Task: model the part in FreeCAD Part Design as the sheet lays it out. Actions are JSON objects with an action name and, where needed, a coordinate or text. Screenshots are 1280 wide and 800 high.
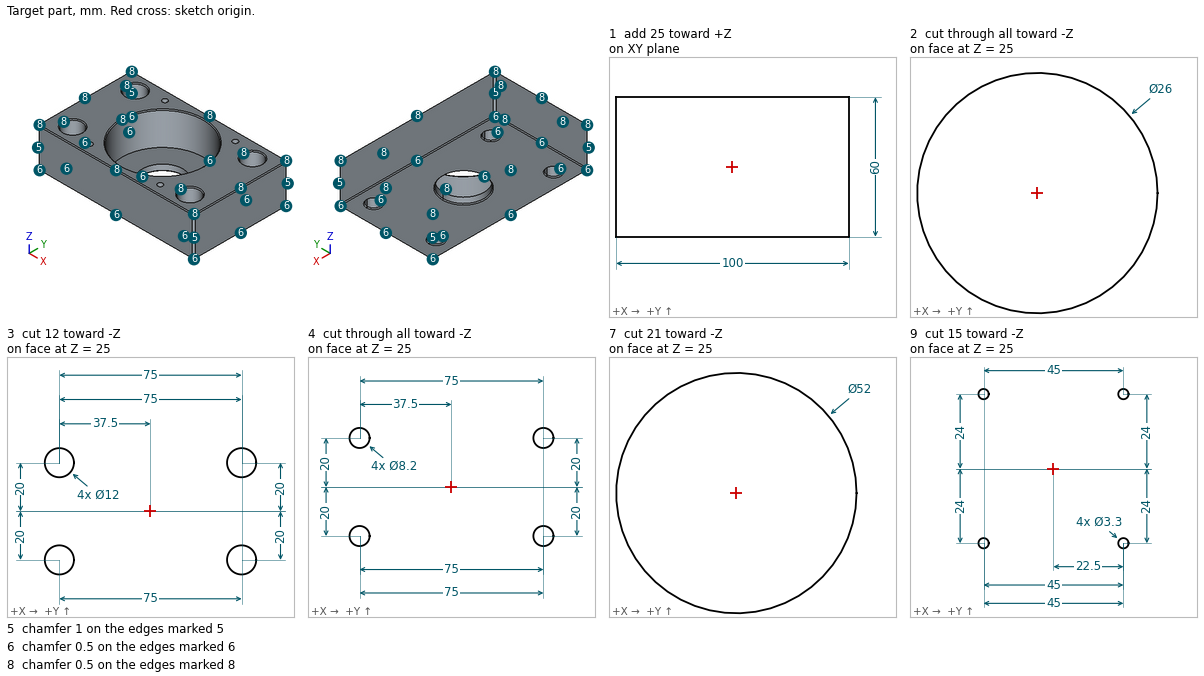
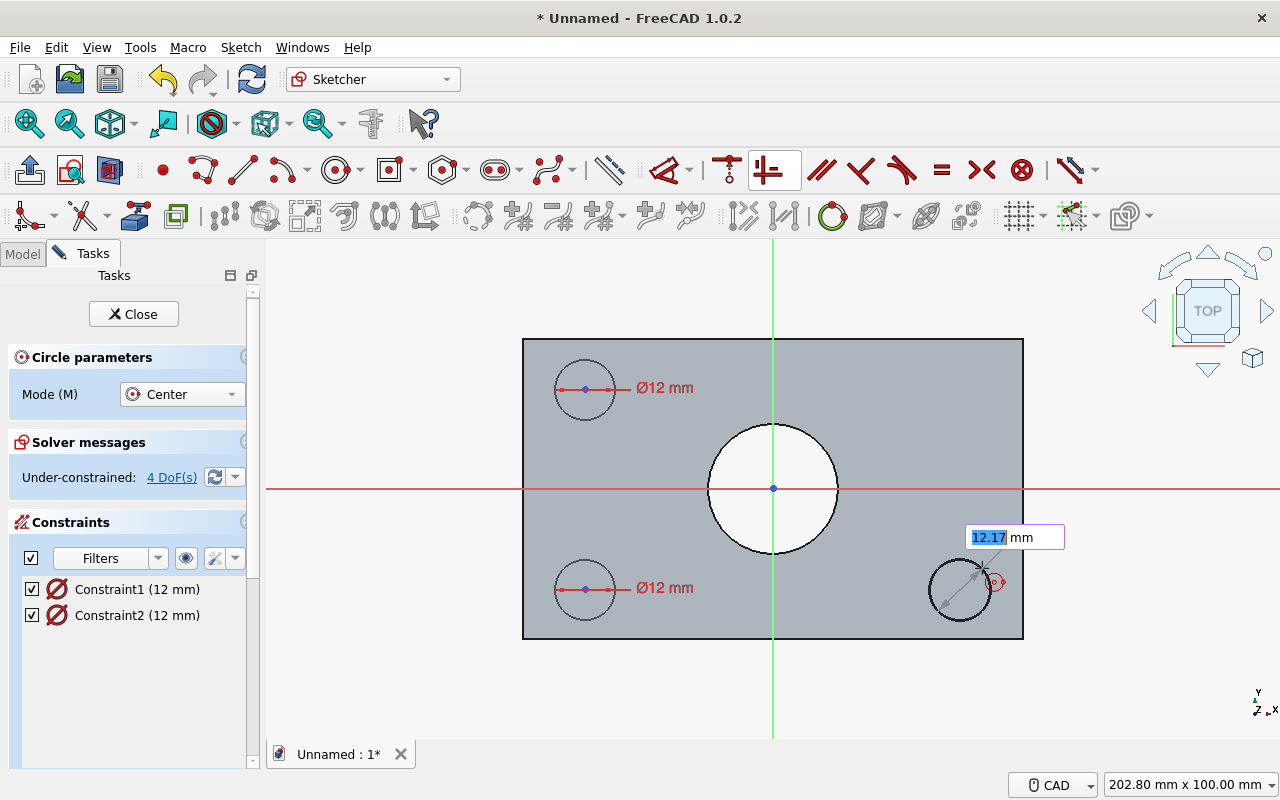
{"action": "type", "text": "12"}
{"action": "key", "text": "Return"}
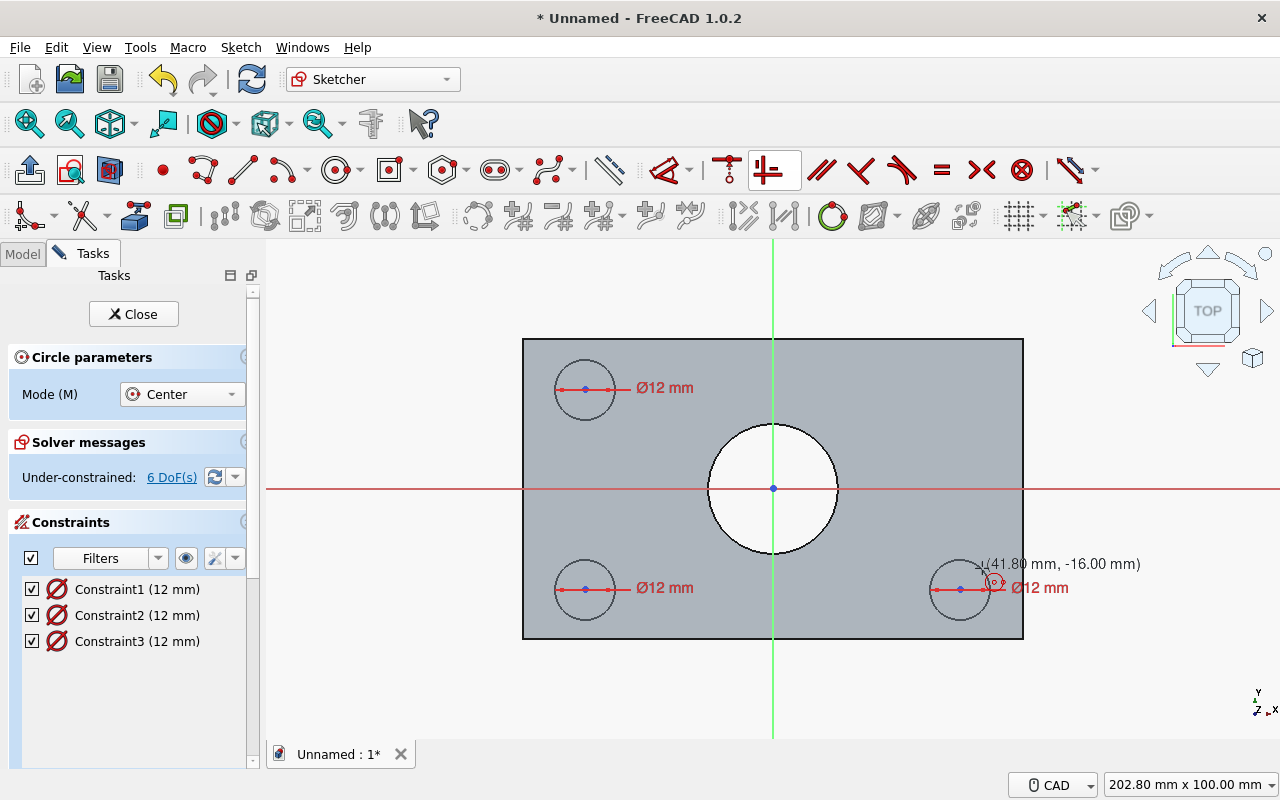
{"action": "left_click", "coordinate": [960, 389]}
{"action": "mouse_move", "coordinate": [982, 368]}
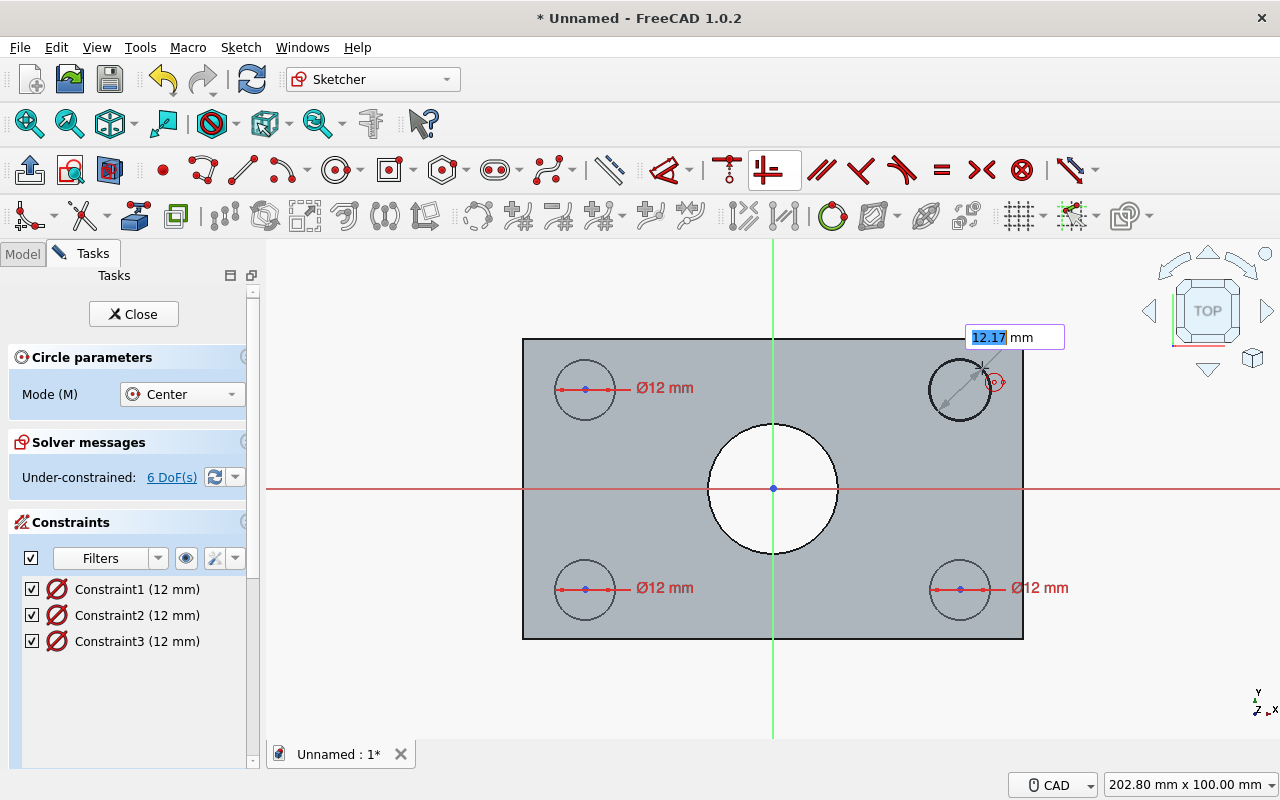
{"action": "type", "text": "12"}
{"action": "key", "text": "Return"}
{"action": "key", "text": "Escape"}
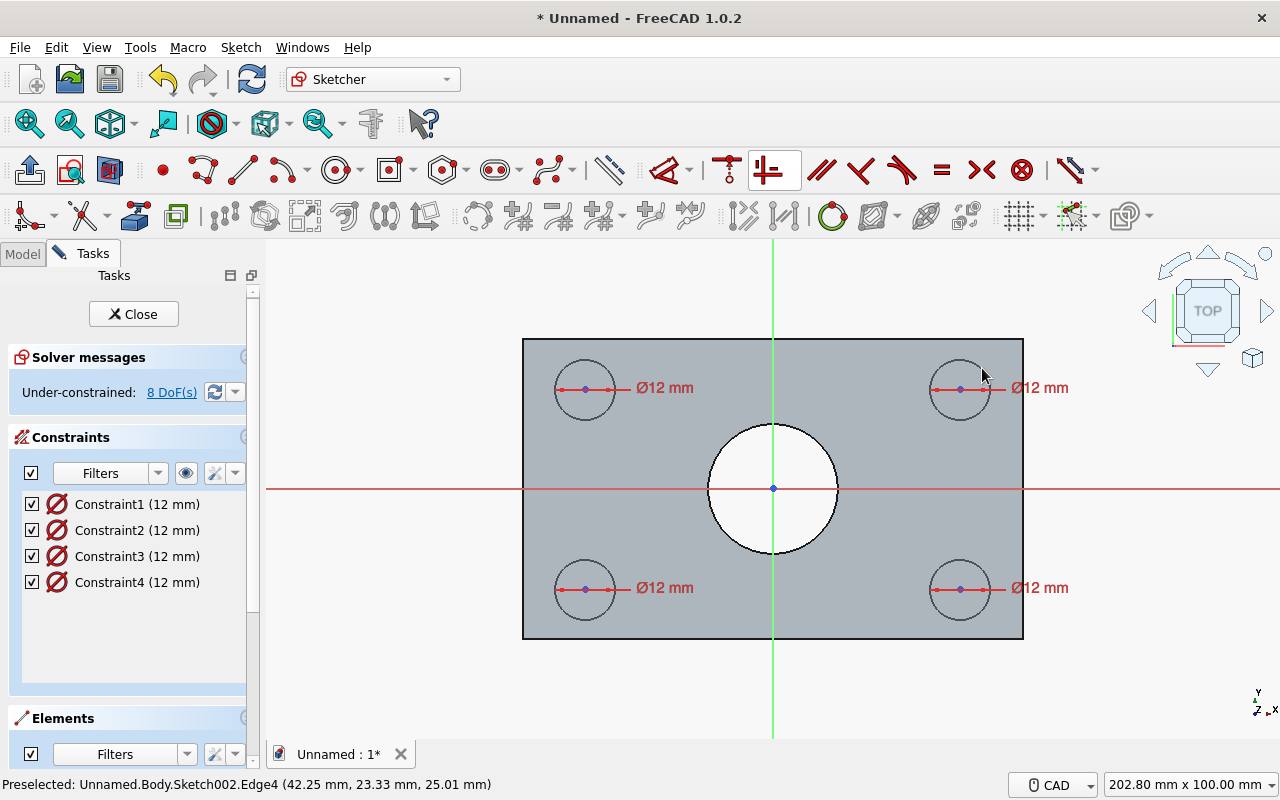
{"action": "left_click", "coordinate": [585, 390]}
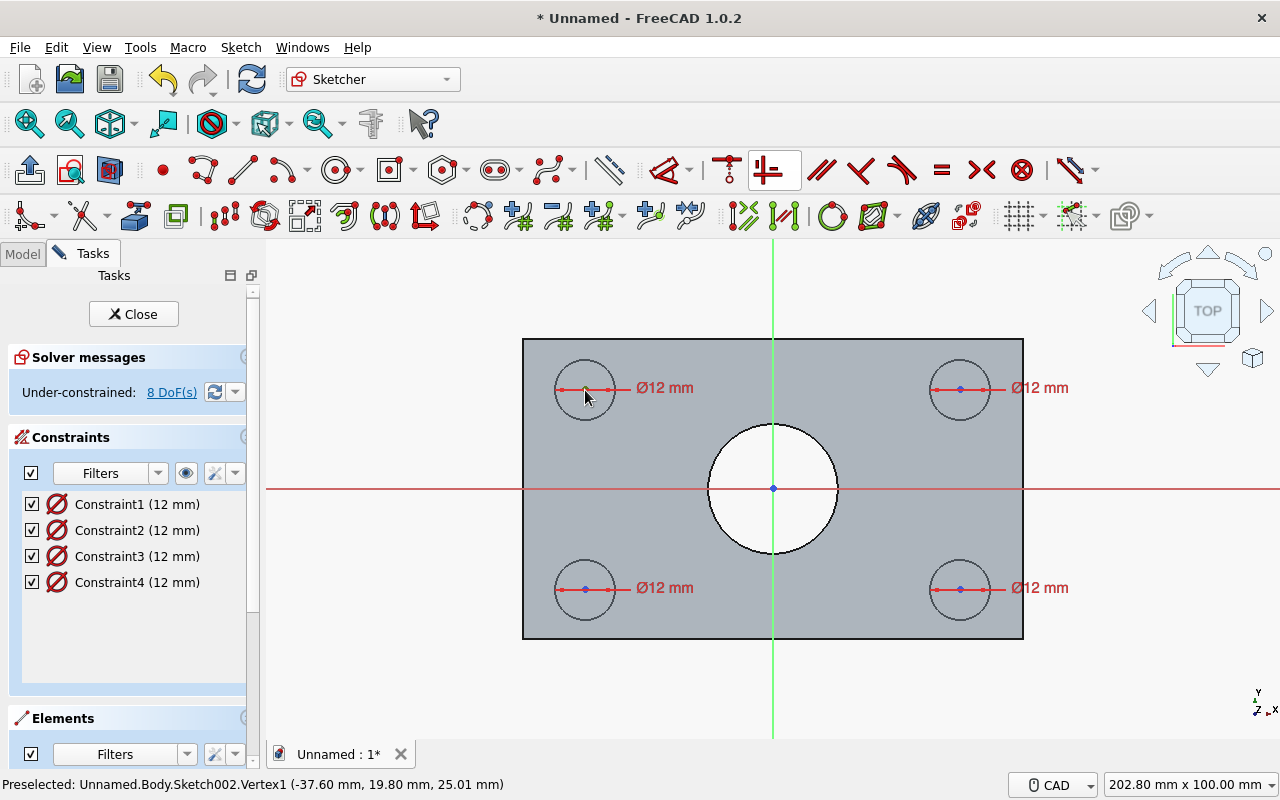
{"action": "key", "text": "i"}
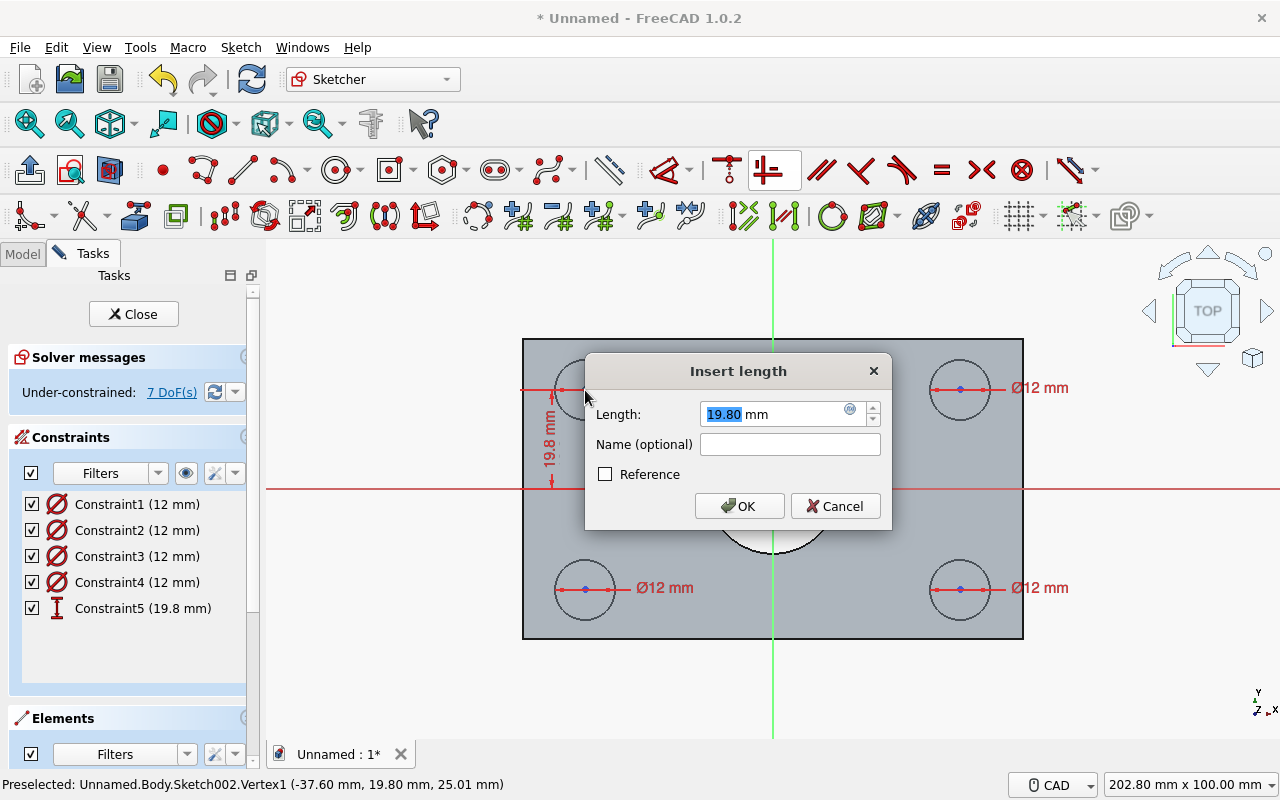
{"action": "type", "text": "20"}
{"action": "key", "text": "Return"}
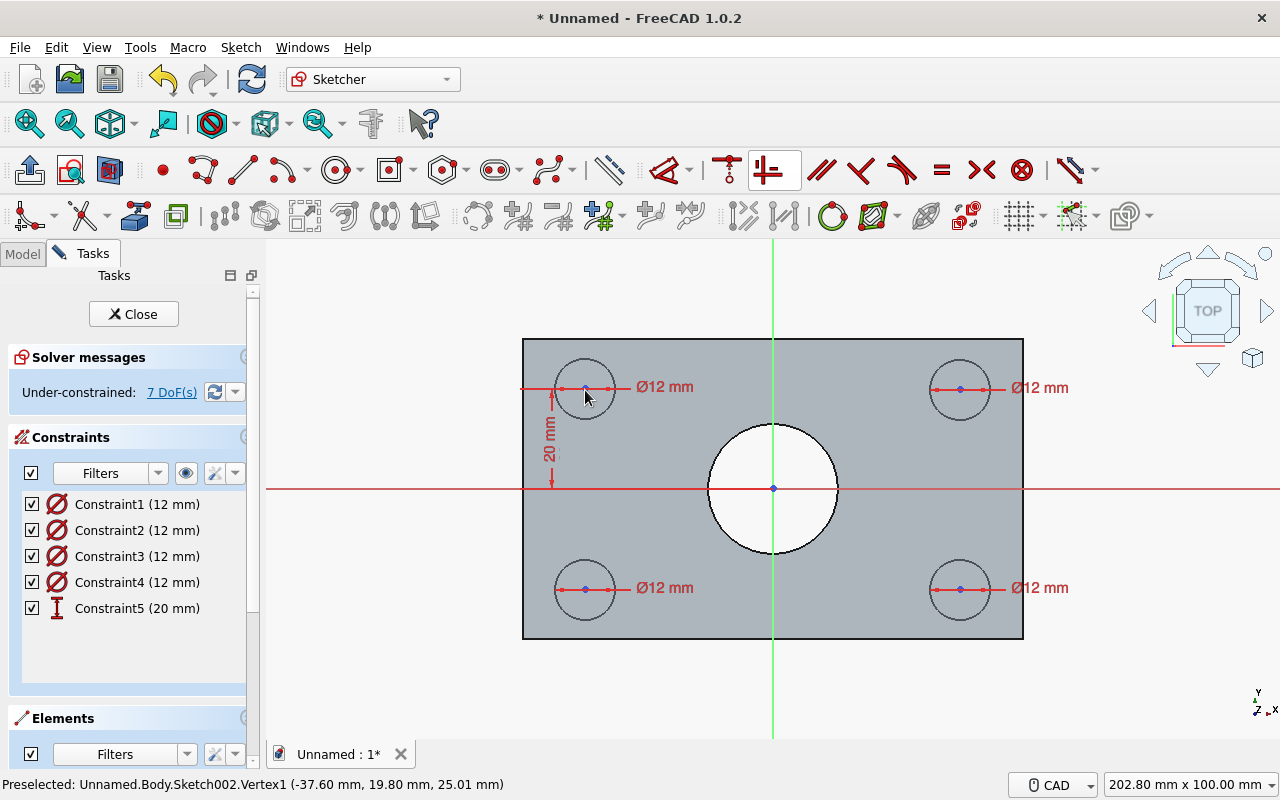
{"action": "left_click", "coordinate": [585, 590]}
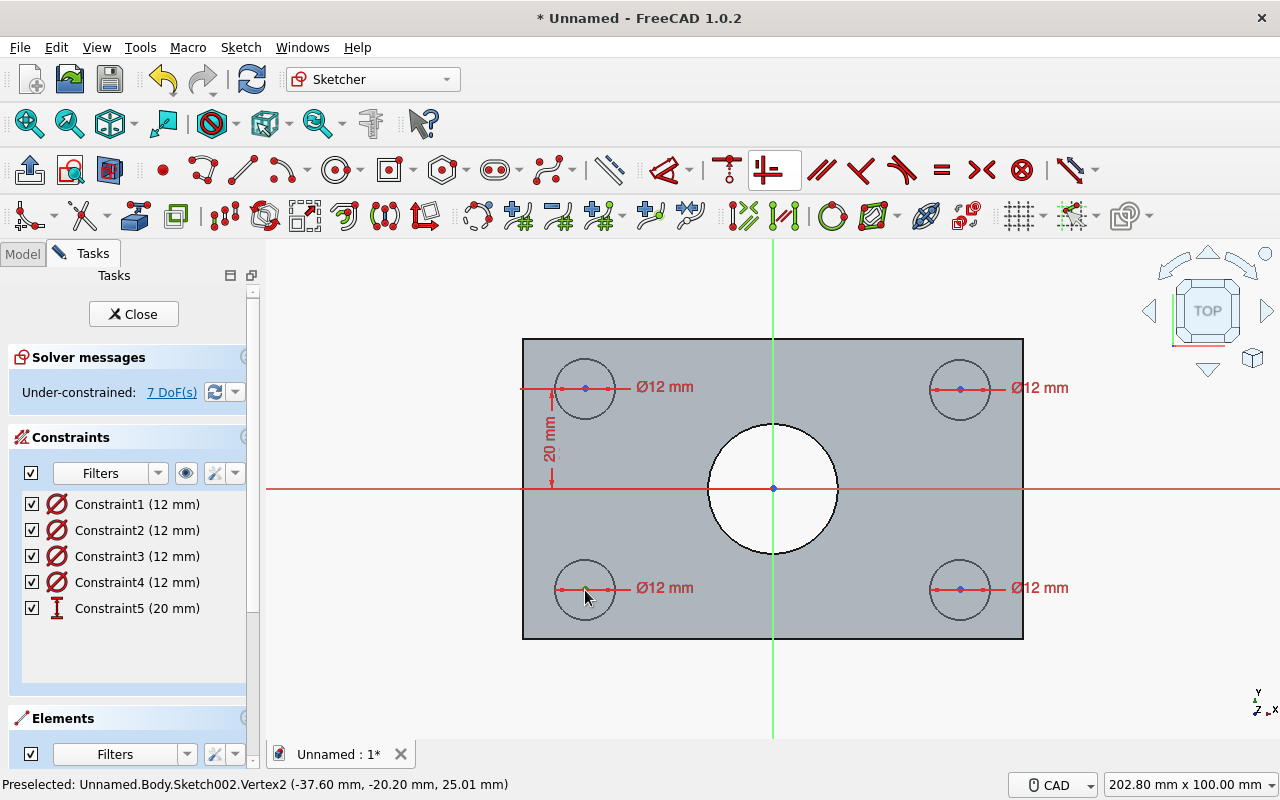
{"action": "key", "text": "i"}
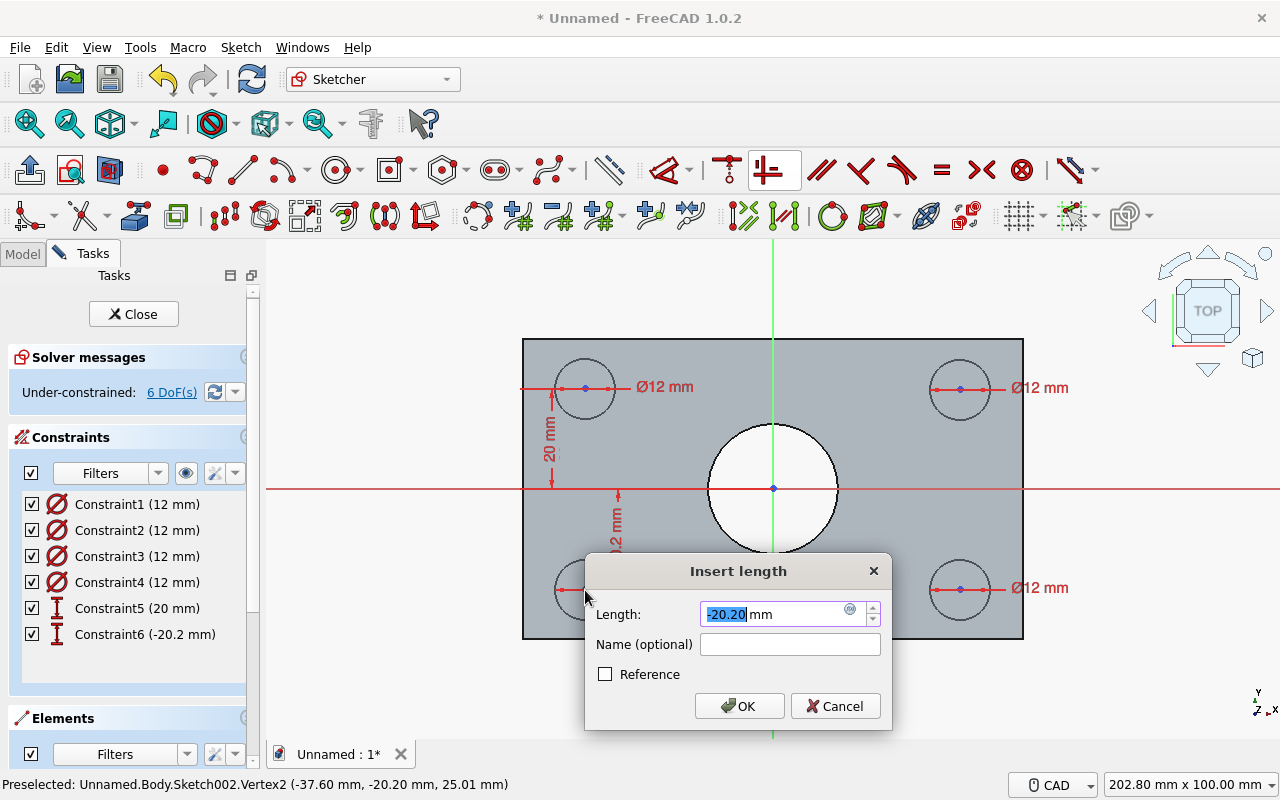
{"action": "type", "text": "-20"}
{"action": "key", "text": "Return"}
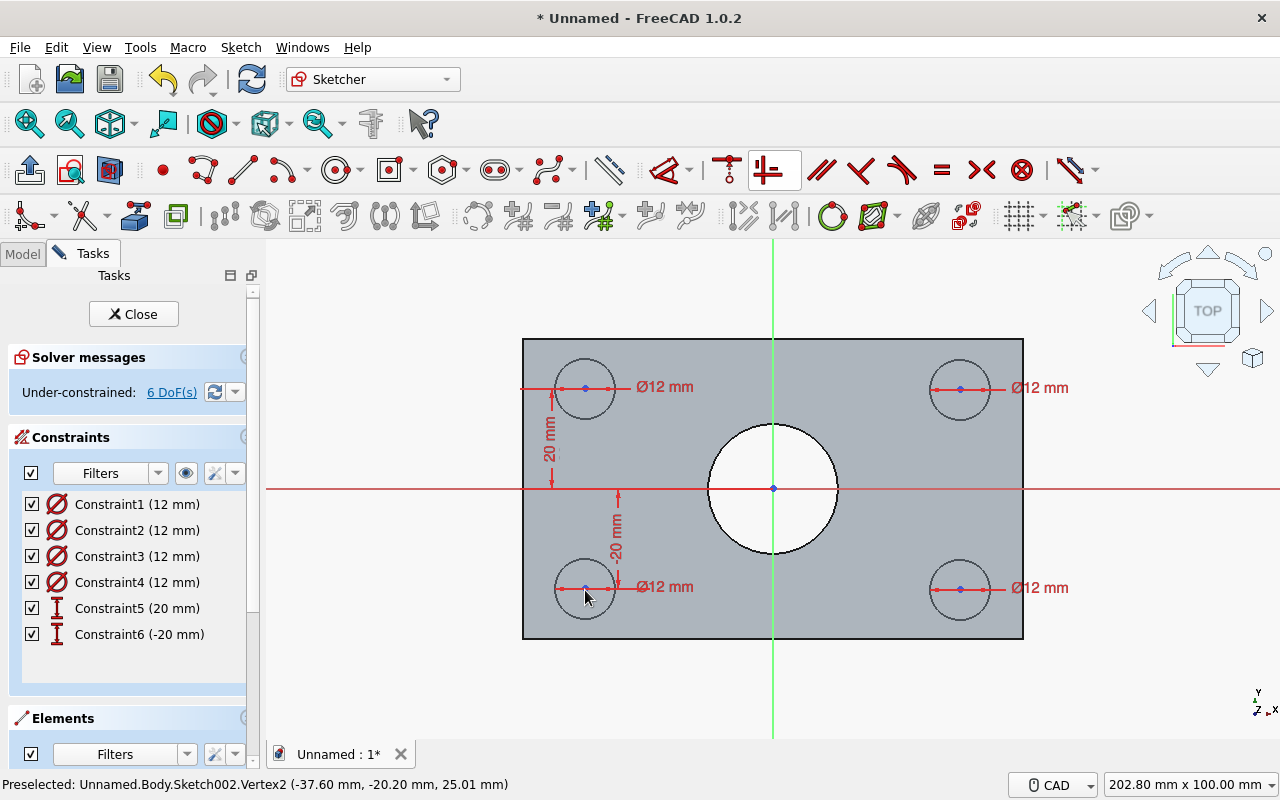
{"action": "left_click", "coordinate": [960, 590]}